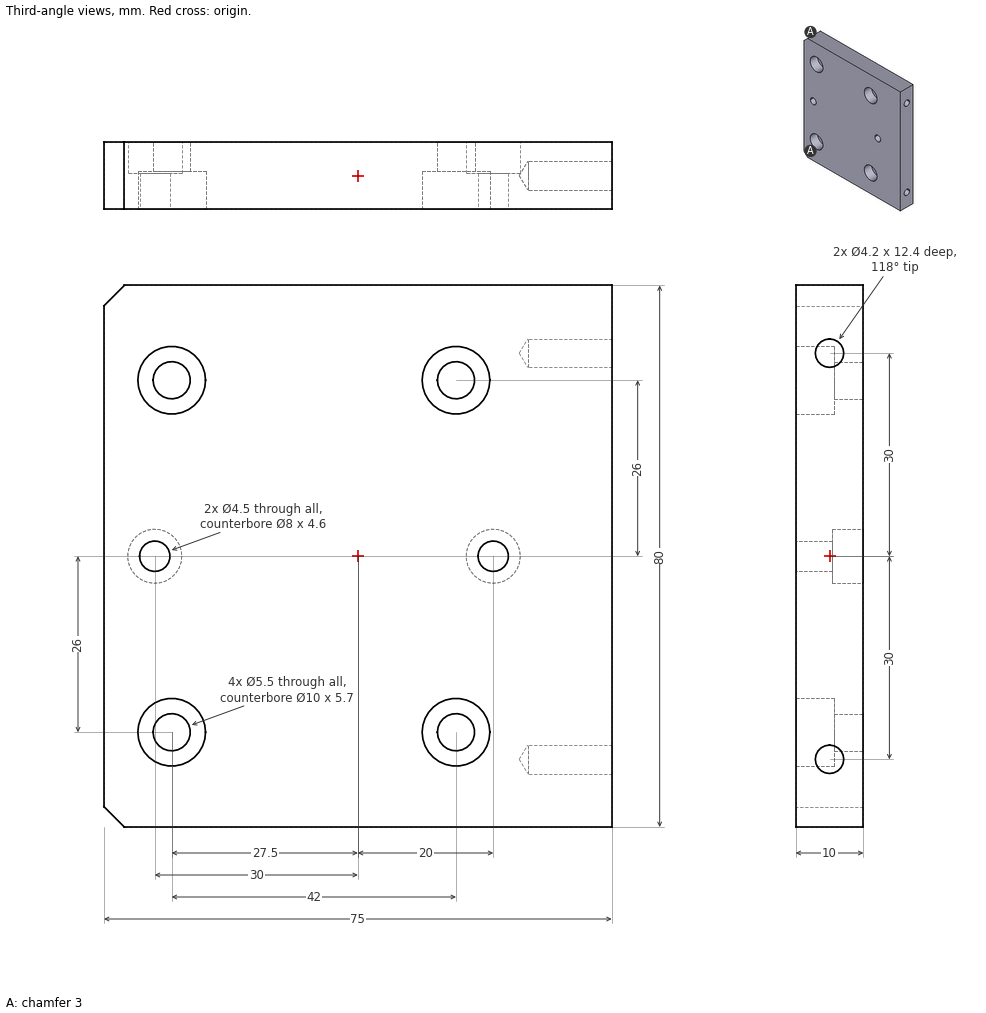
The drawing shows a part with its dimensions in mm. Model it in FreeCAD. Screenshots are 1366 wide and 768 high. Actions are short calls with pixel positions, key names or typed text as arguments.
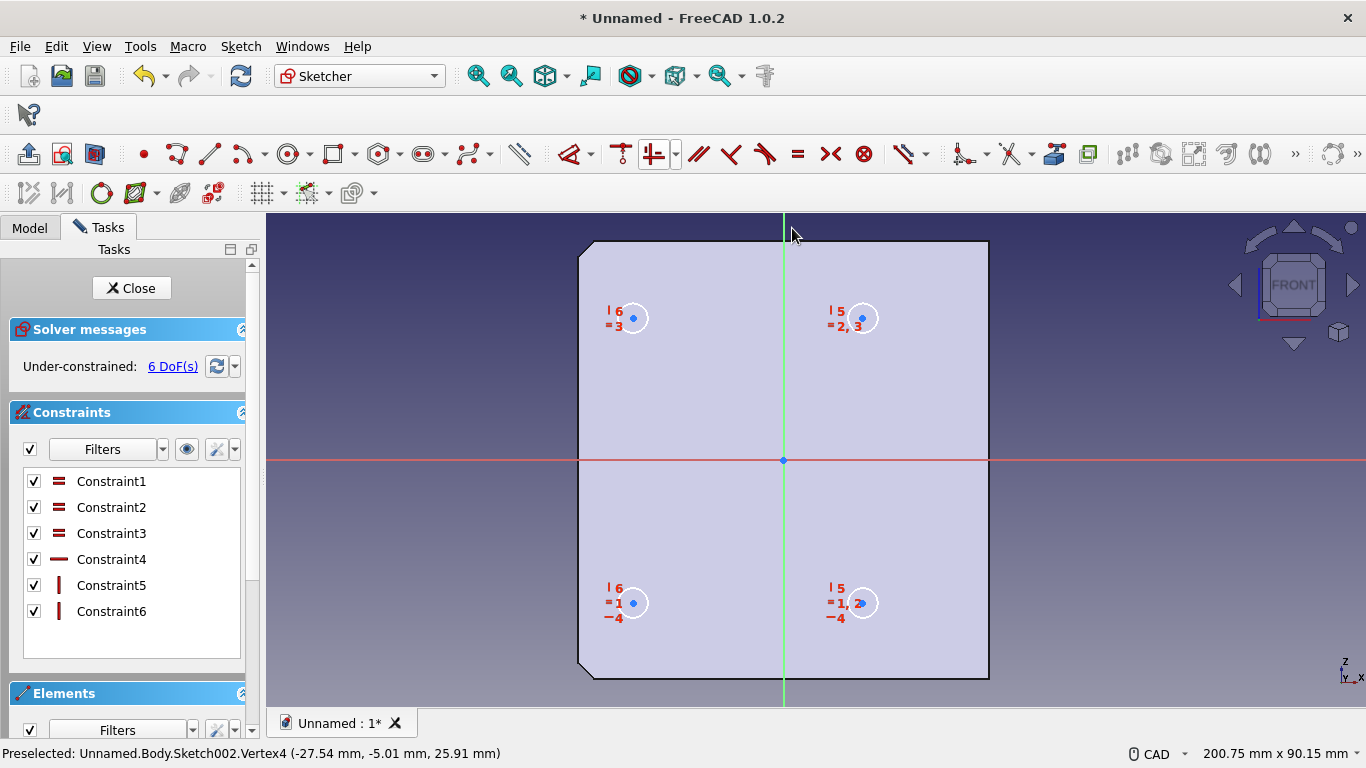
click(863, 318)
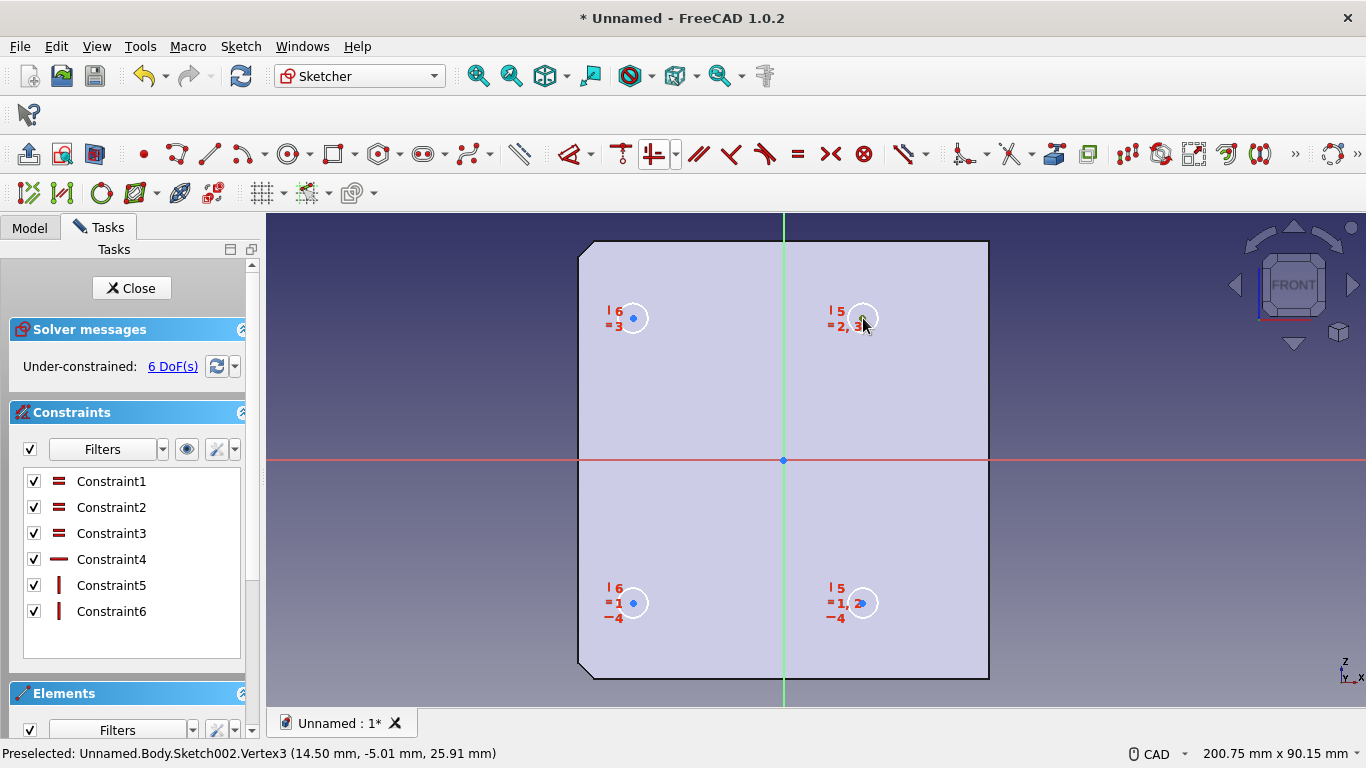
click(633, 318)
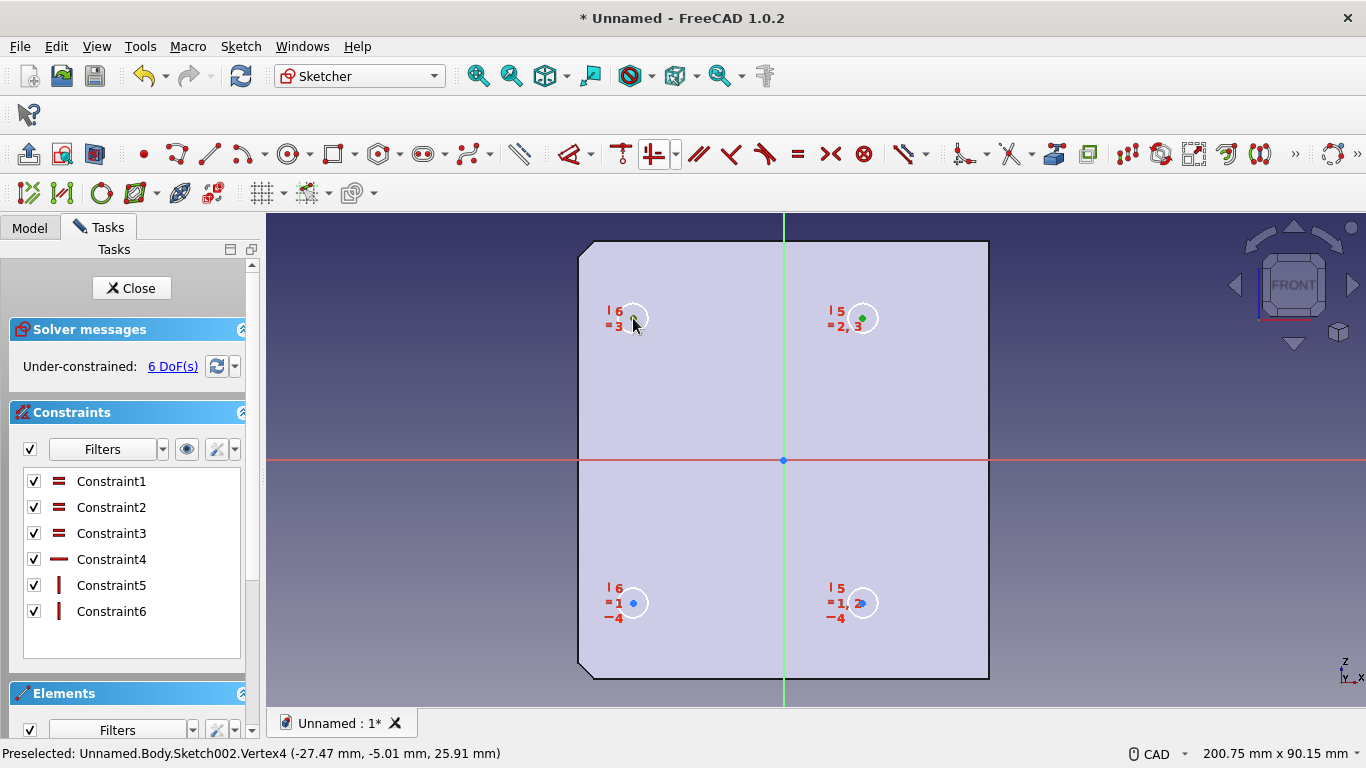
click(676, 154)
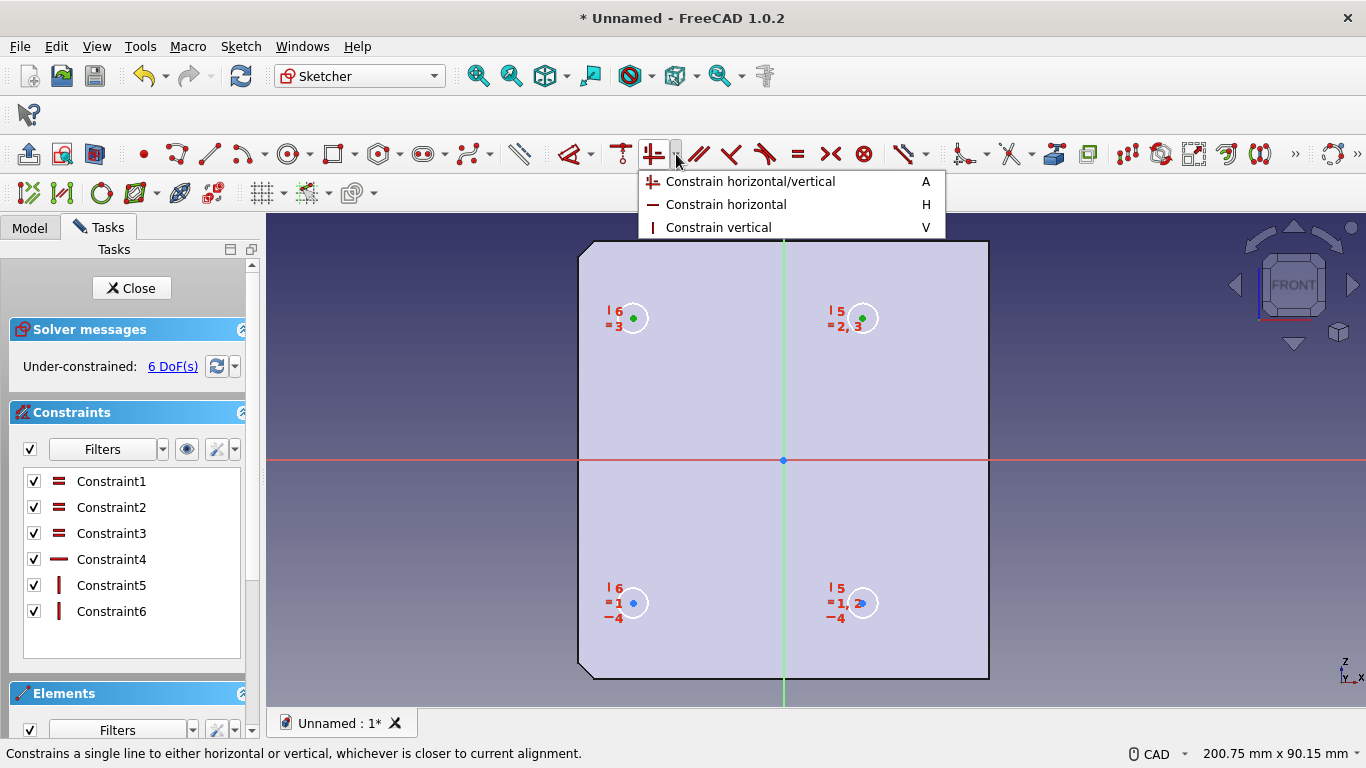
click(792, 204)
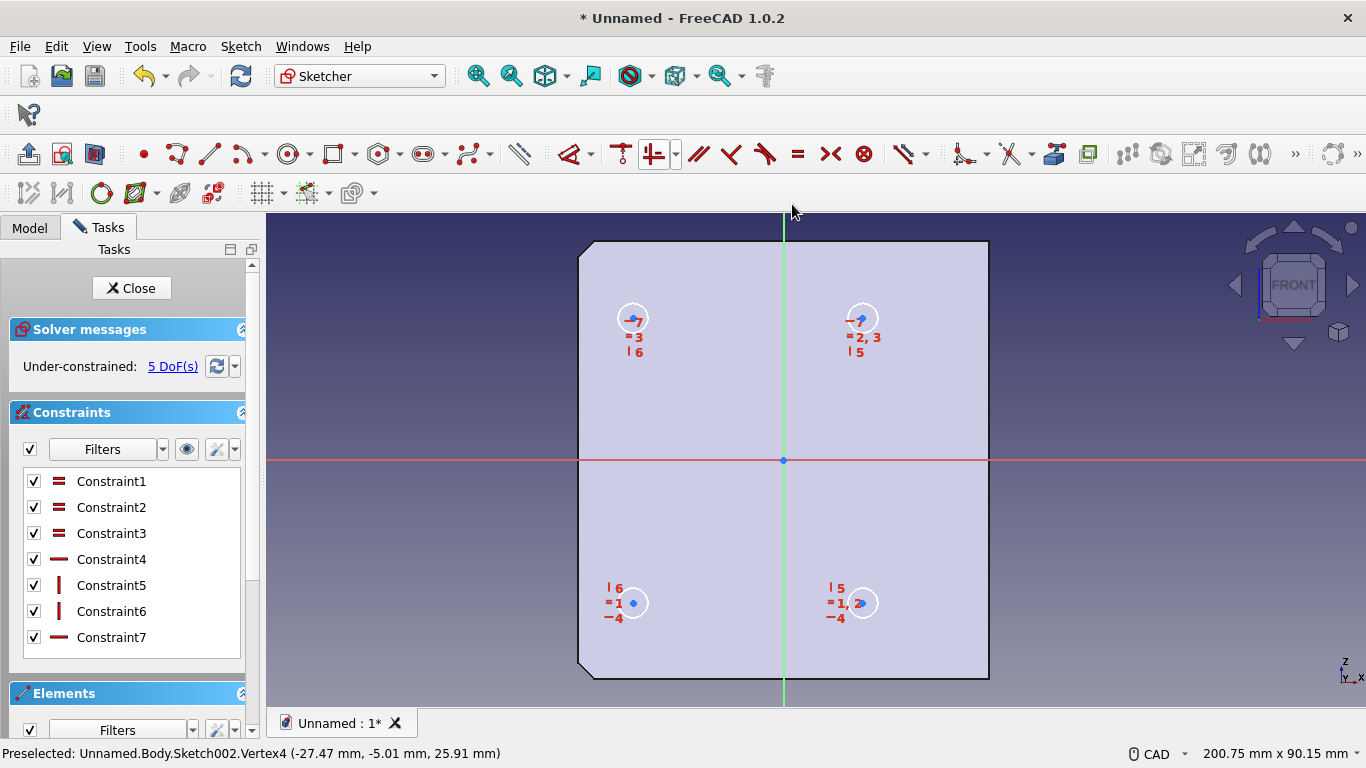
key(d)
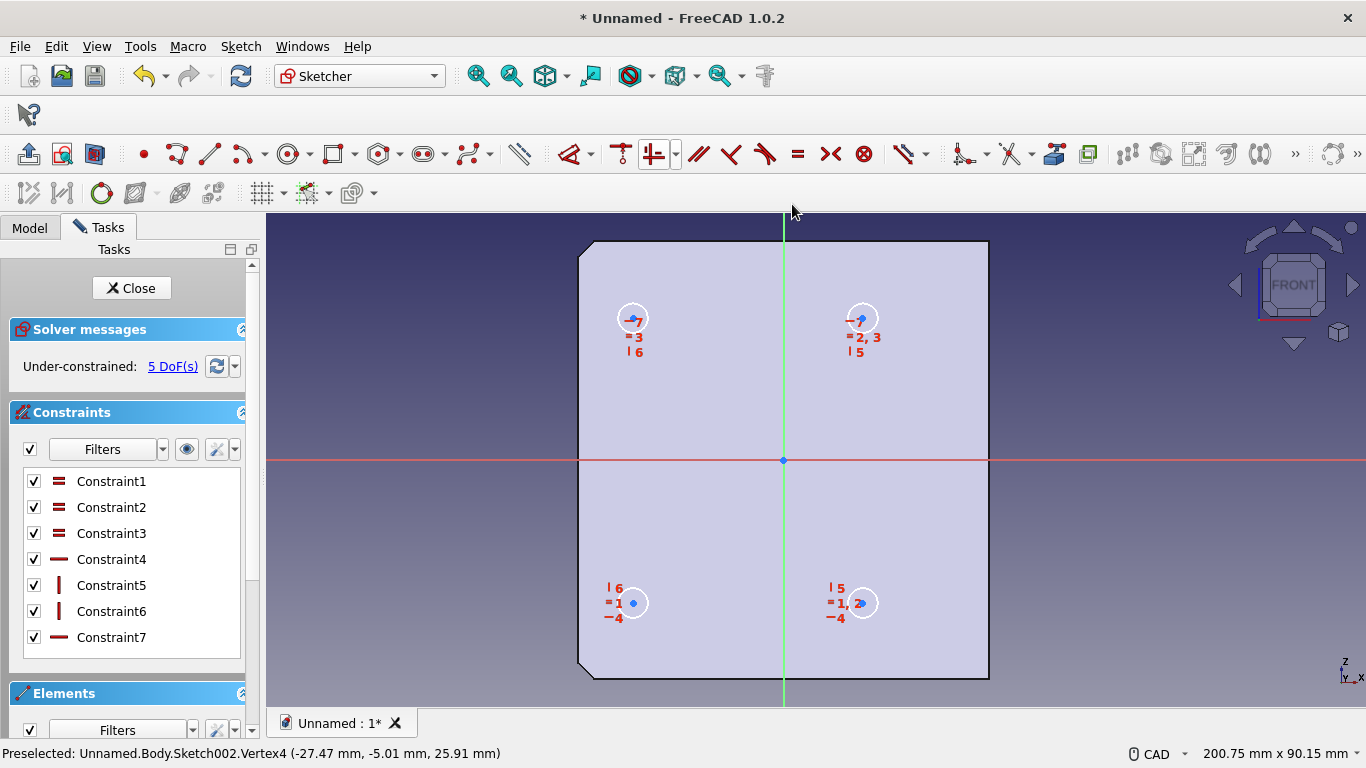
scroll(643, 593, up, 2)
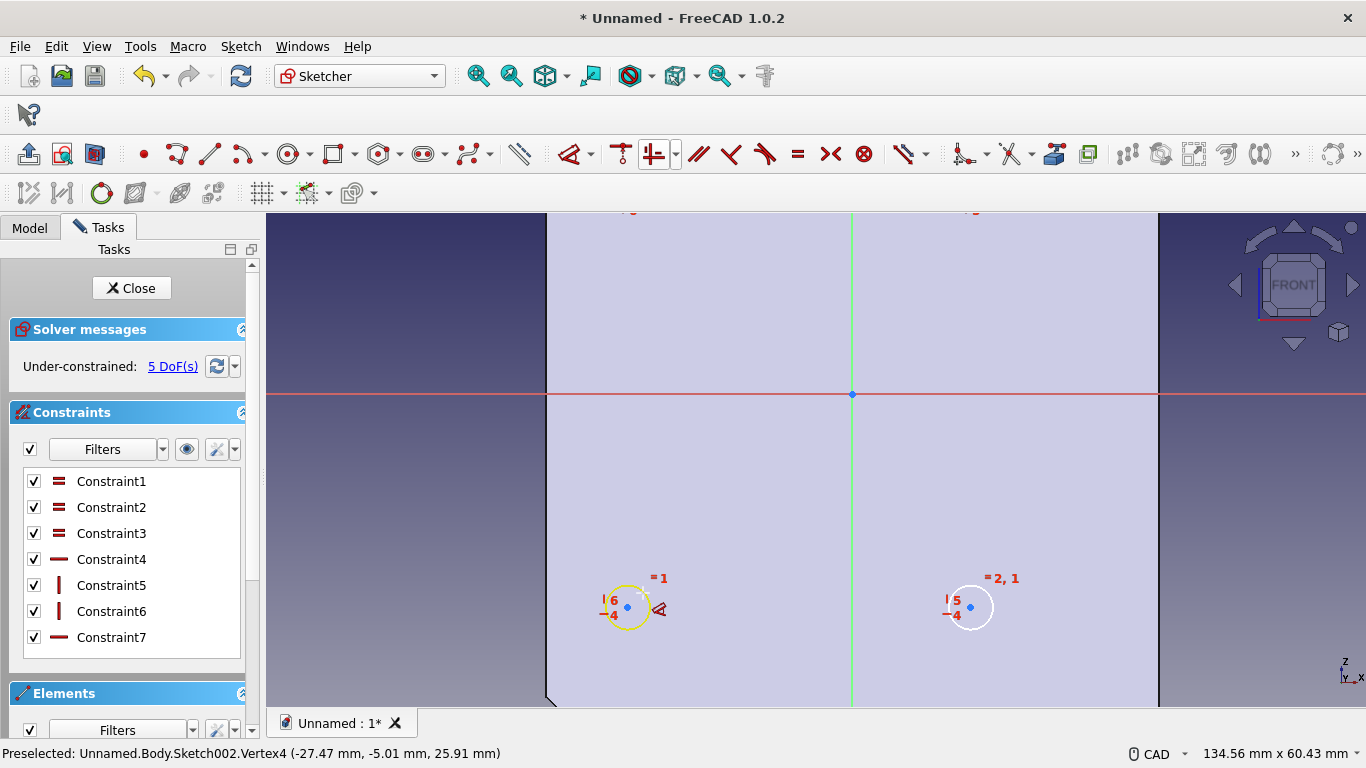
click(643, 592)
click(665, 569)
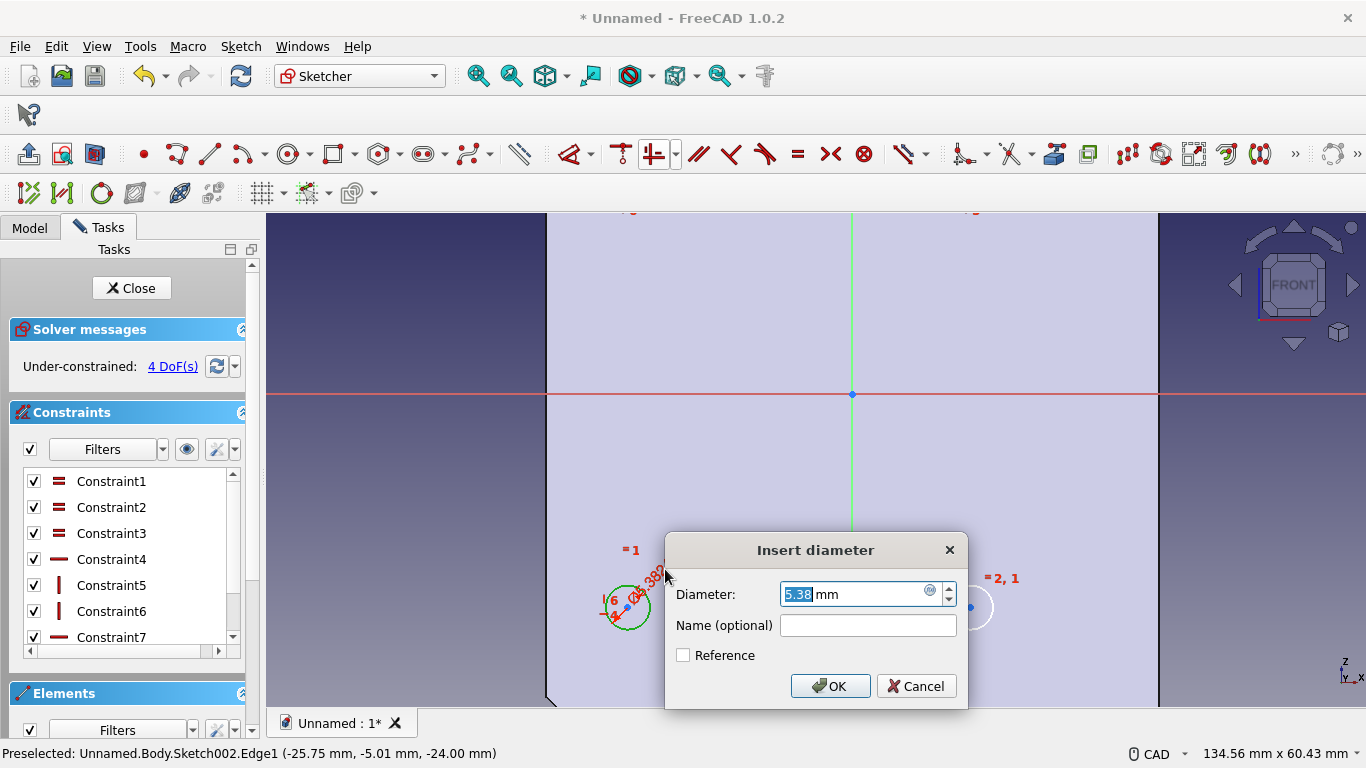
text(5.5)
key(Return)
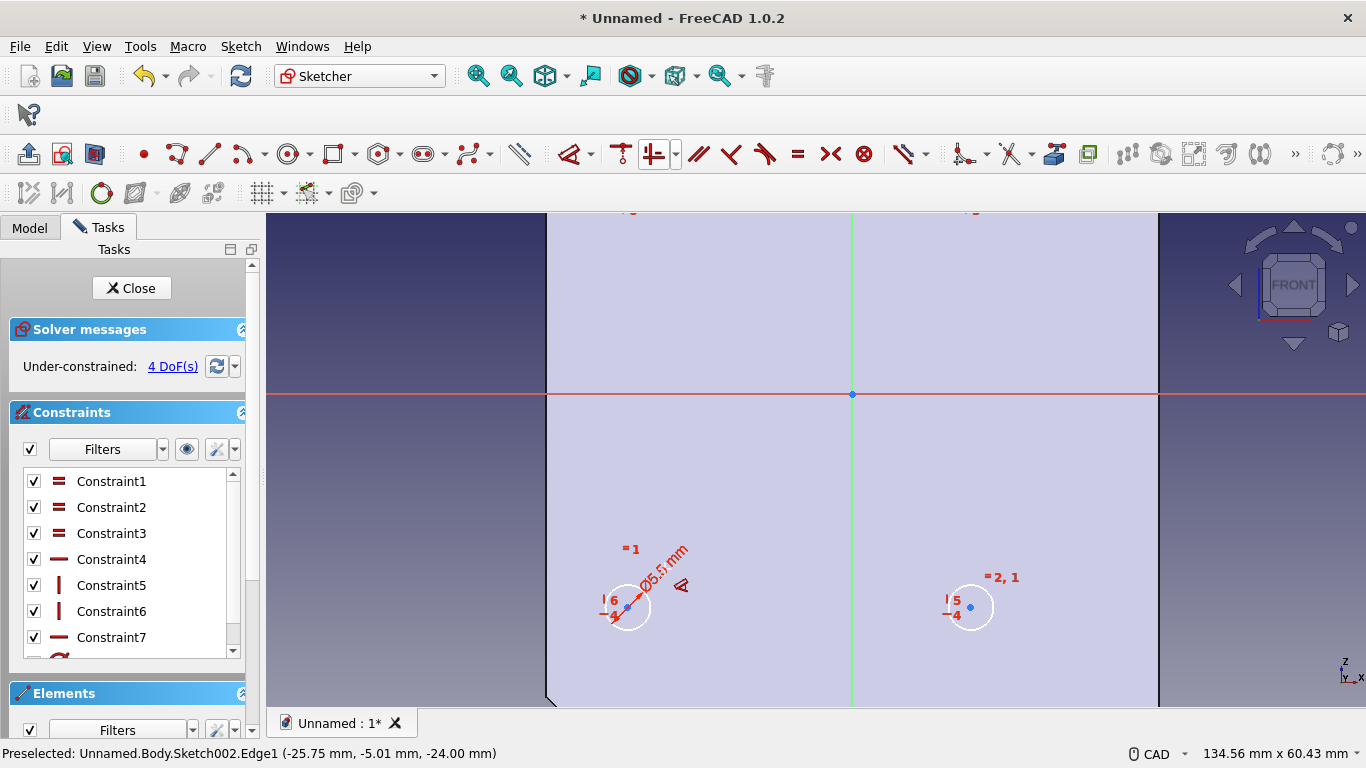
click(628, 608)
click(594, 501)